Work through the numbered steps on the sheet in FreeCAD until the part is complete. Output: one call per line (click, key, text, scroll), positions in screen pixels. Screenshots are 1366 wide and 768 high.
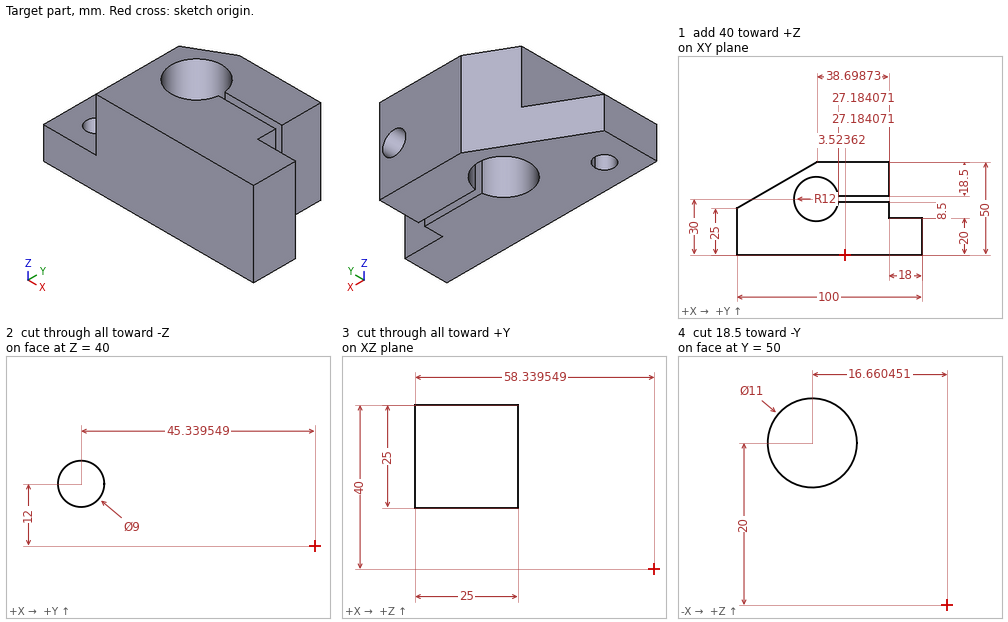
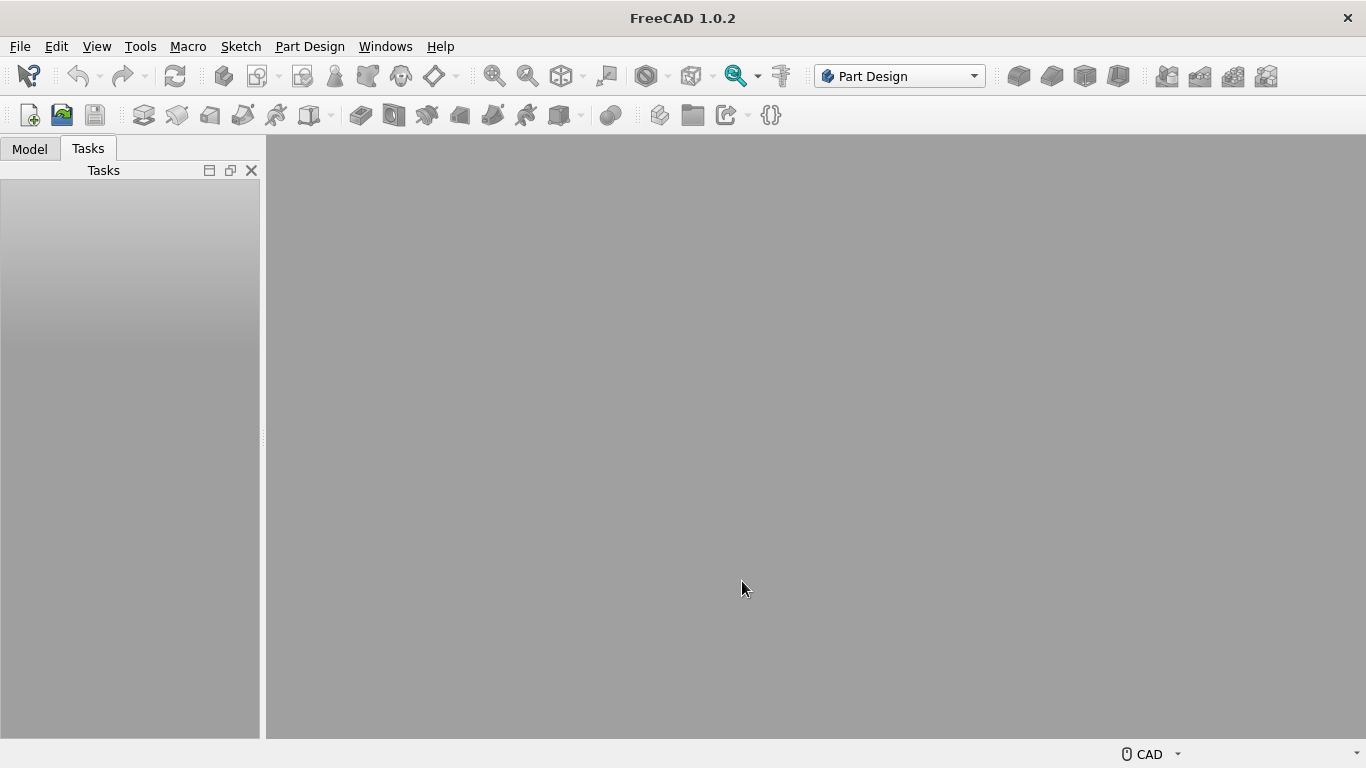
key(ctrl+n)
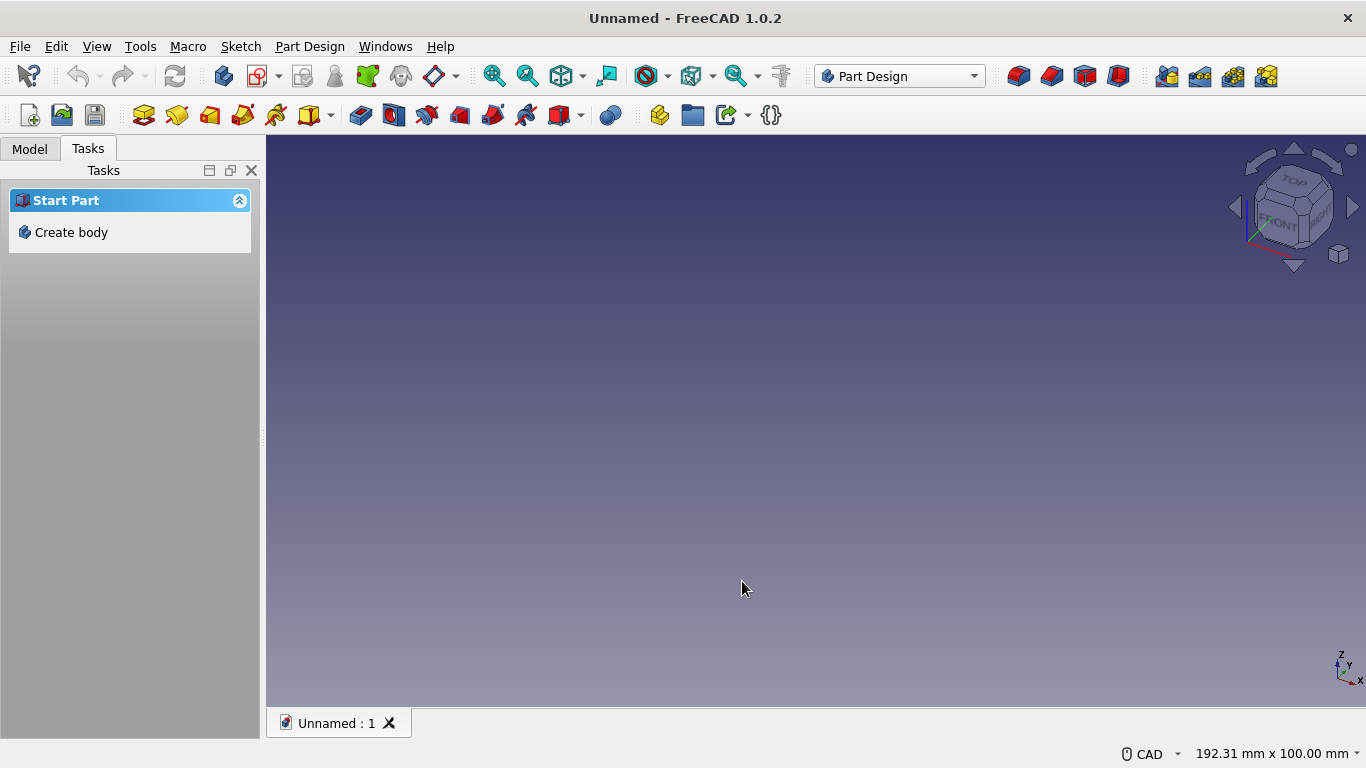
click(256, 76)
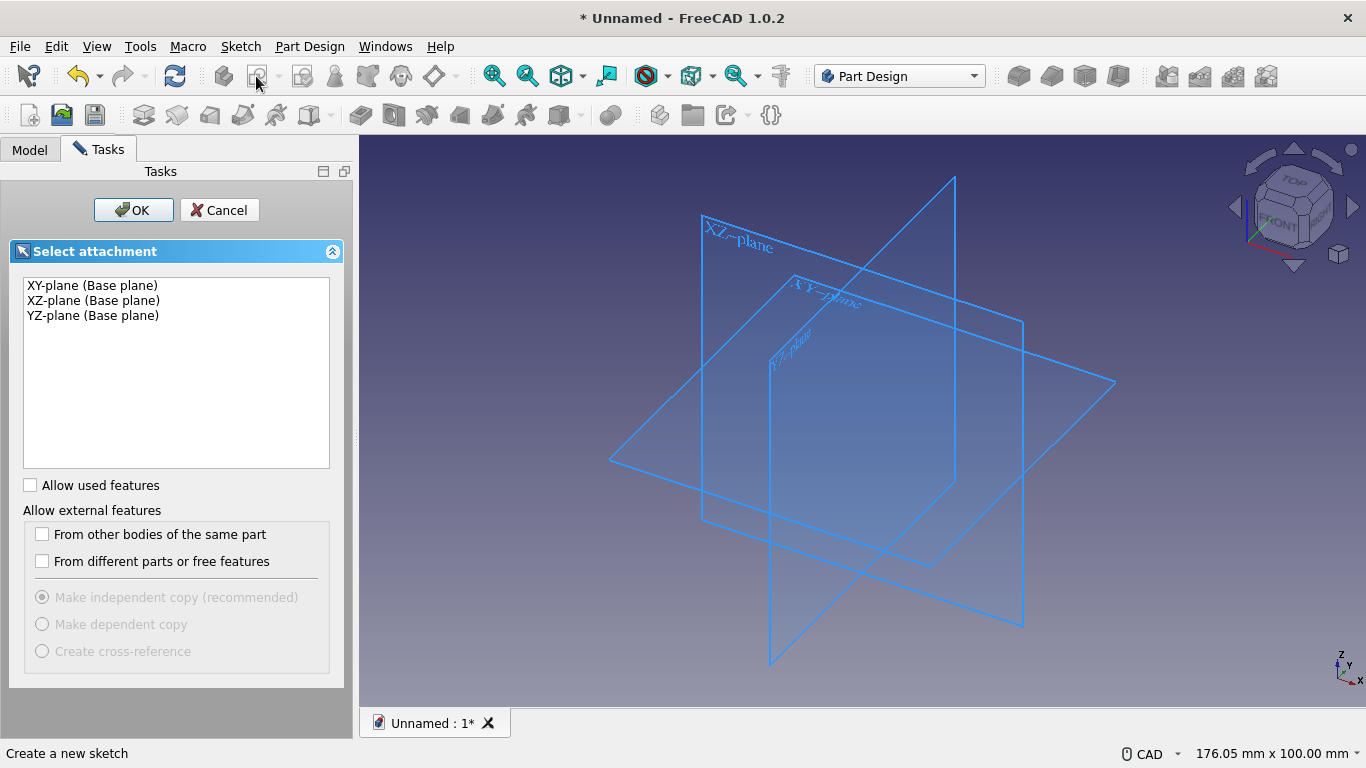
click(84, 286)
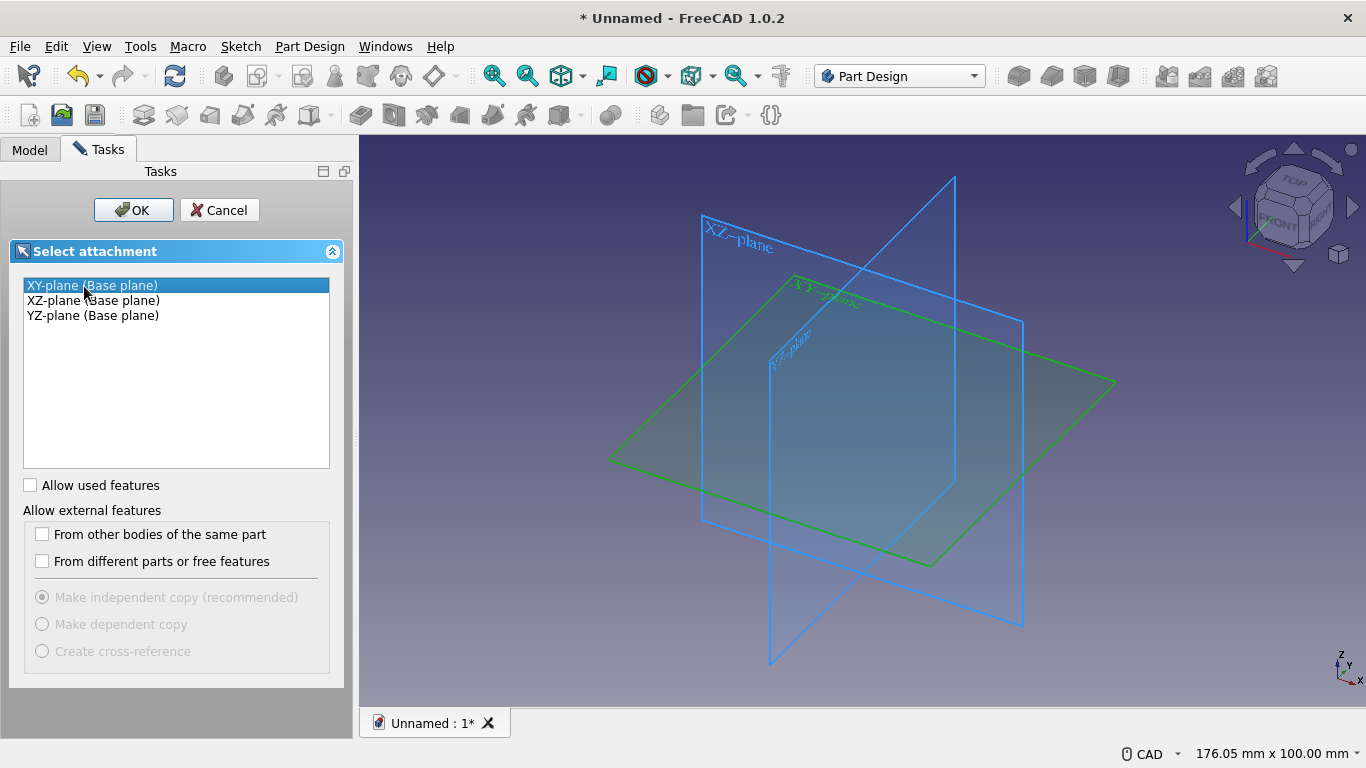
click(134, 210)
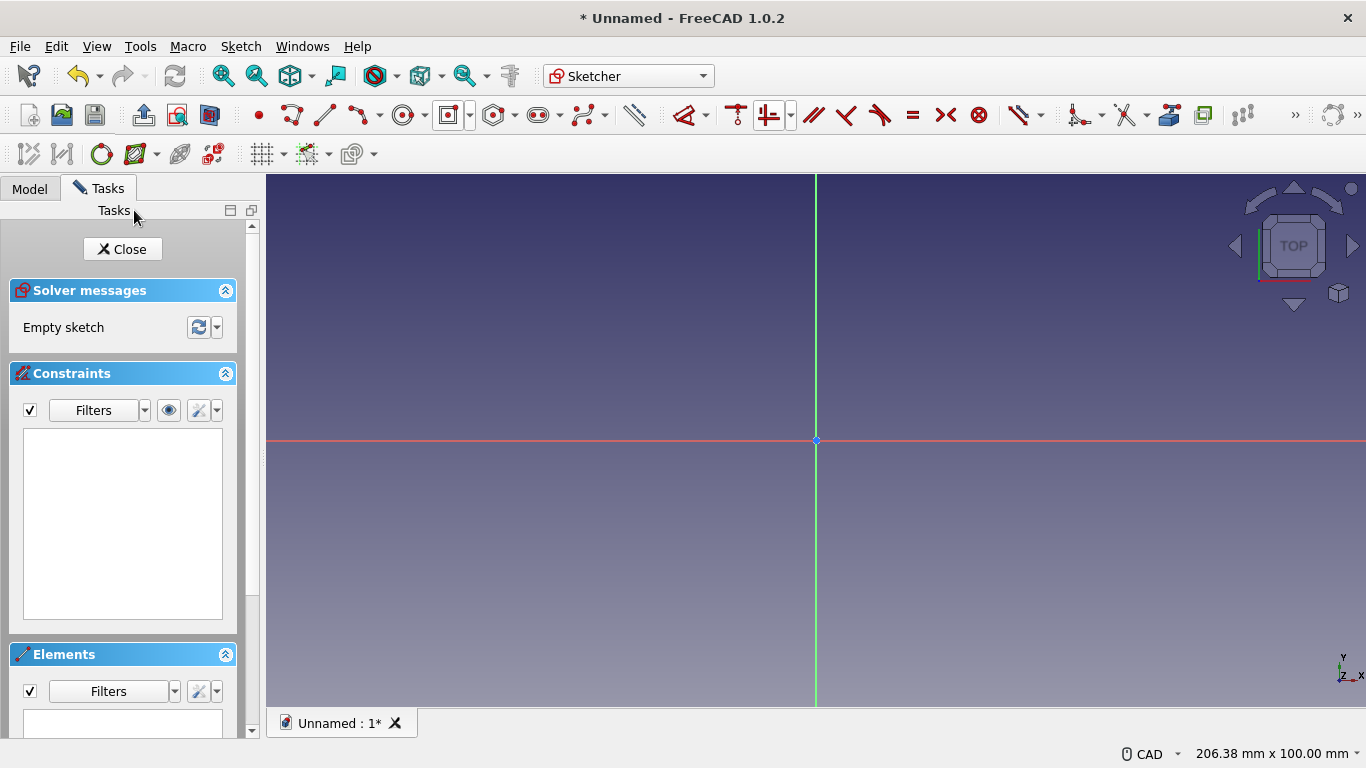
scroll(639, 679, down, 1)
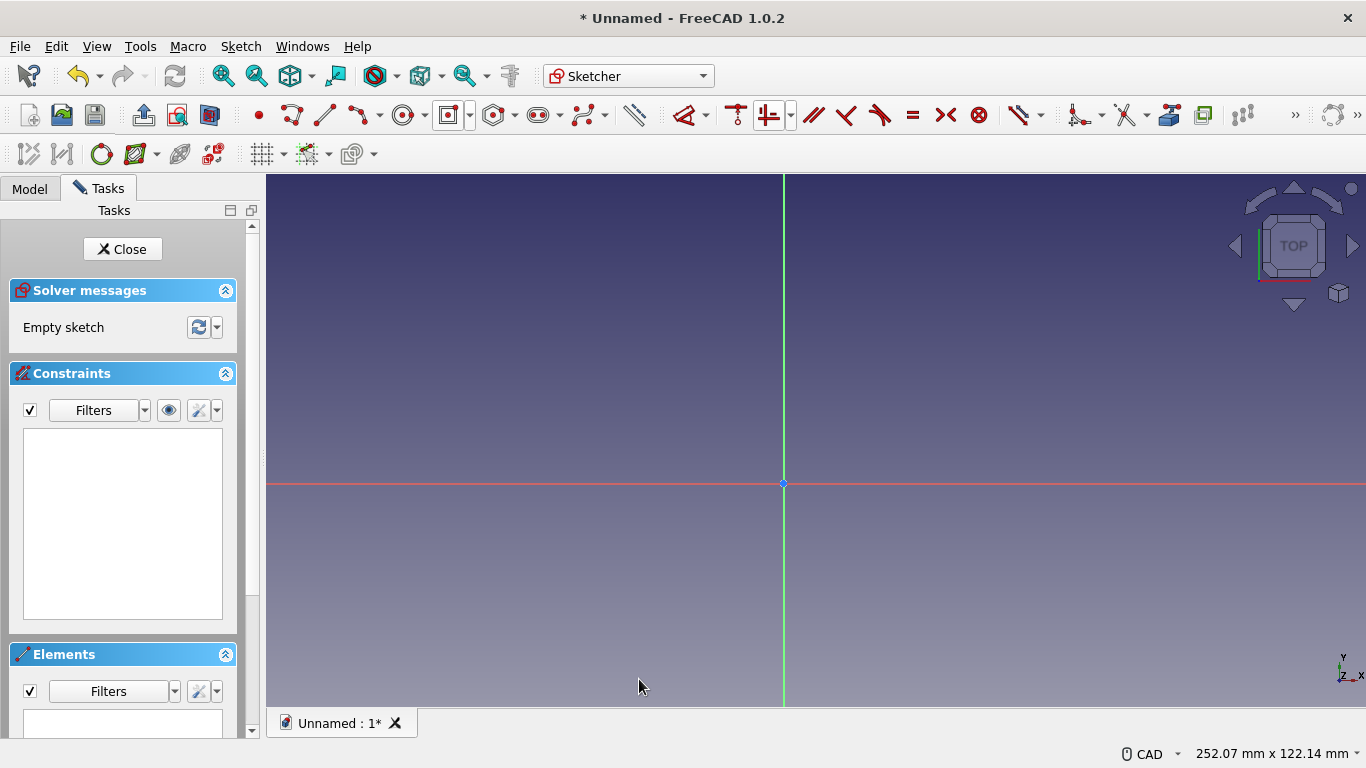
scroll(748, 241, up, 2)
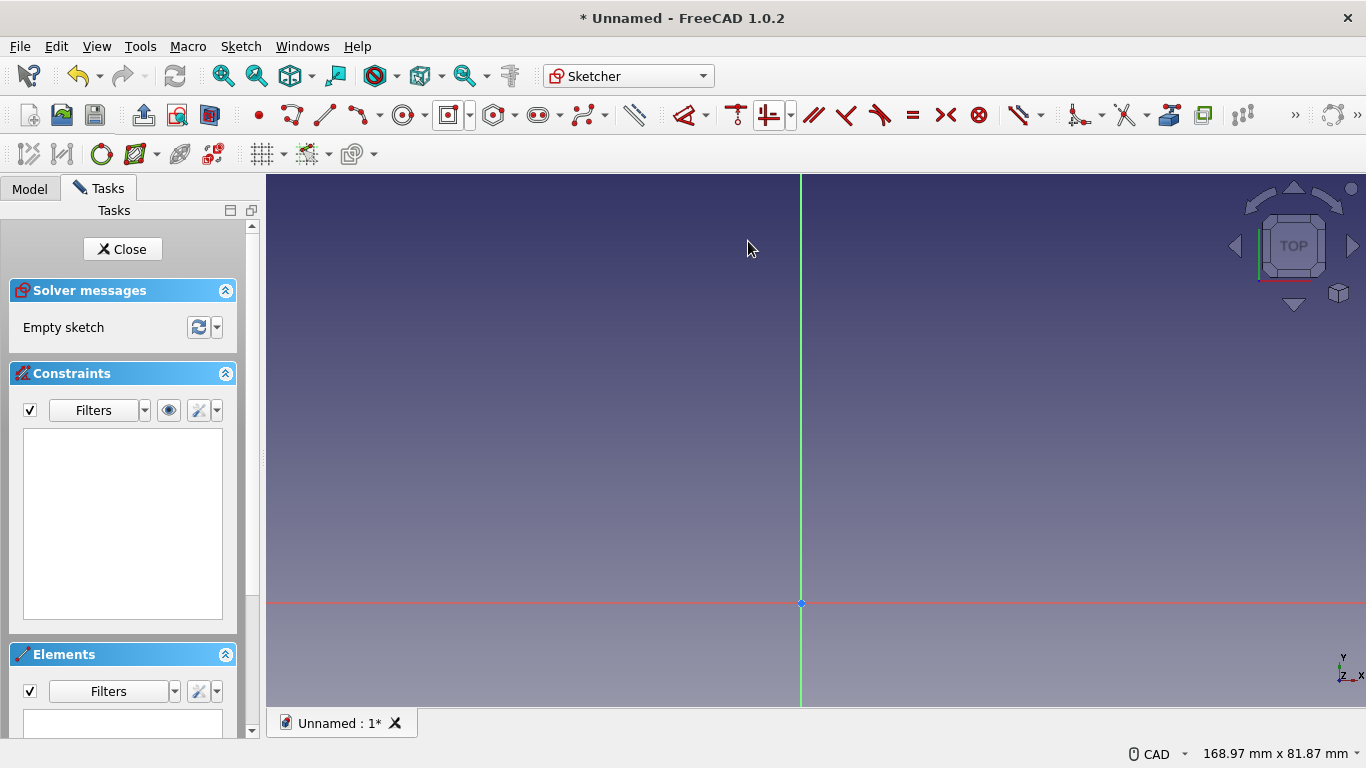
click(292, 116)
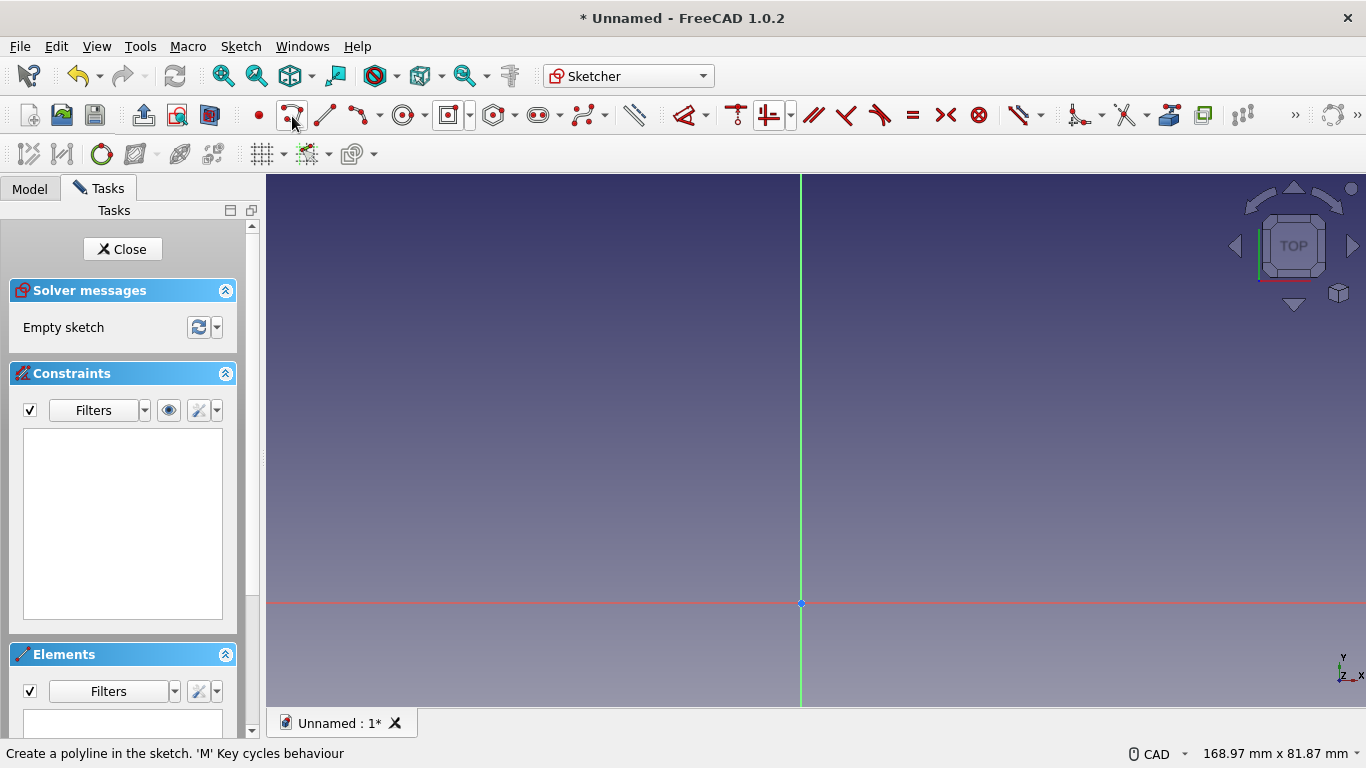
click(779, 398)
click(955, 398)
click(955, 278)
click(704, 278)
click(422, 441)
click(422, 603)
click(1073, 594)
click(1073, 473)
click(955, 473)
click(955, 418)
click(779, 418)
right_click(779, 418)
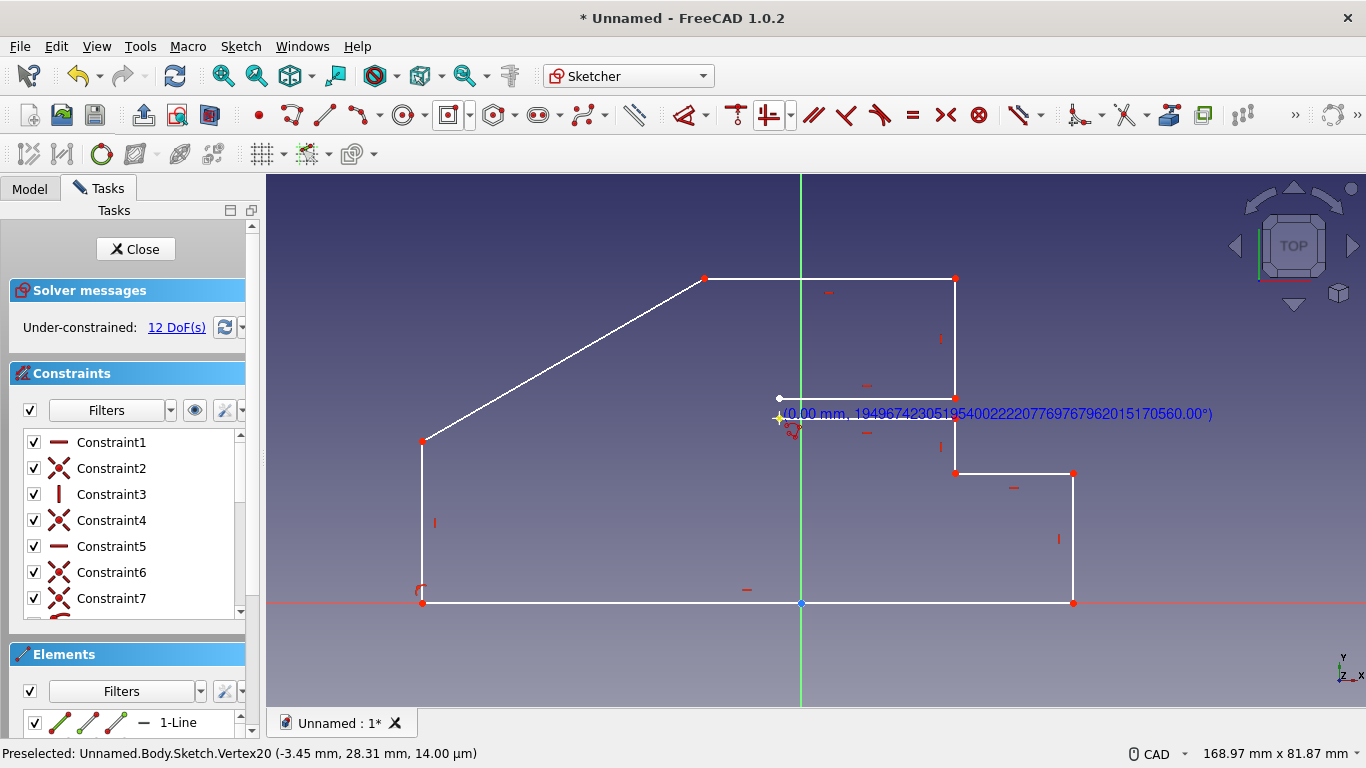
click(358, 116)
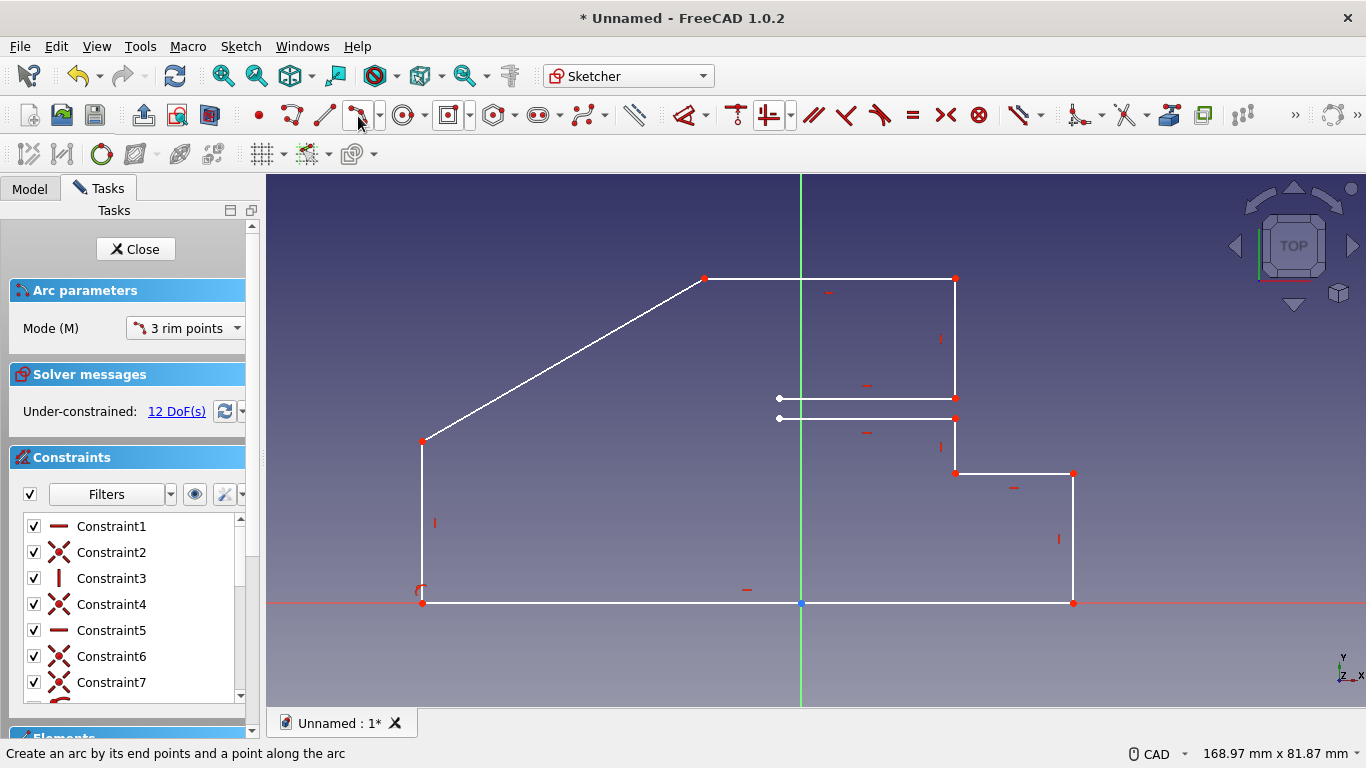
click(779, 419)
click(779, 399)
click(623, 408)
key(Escape)